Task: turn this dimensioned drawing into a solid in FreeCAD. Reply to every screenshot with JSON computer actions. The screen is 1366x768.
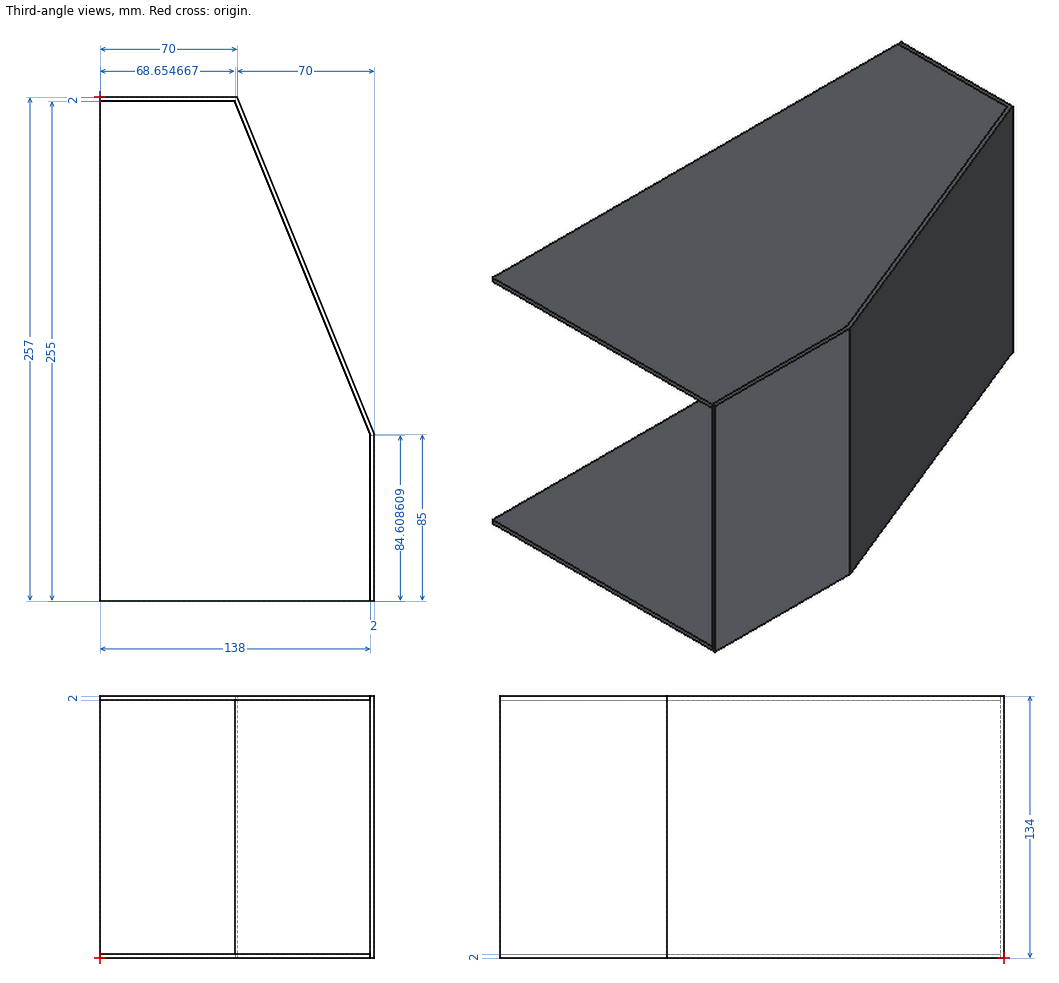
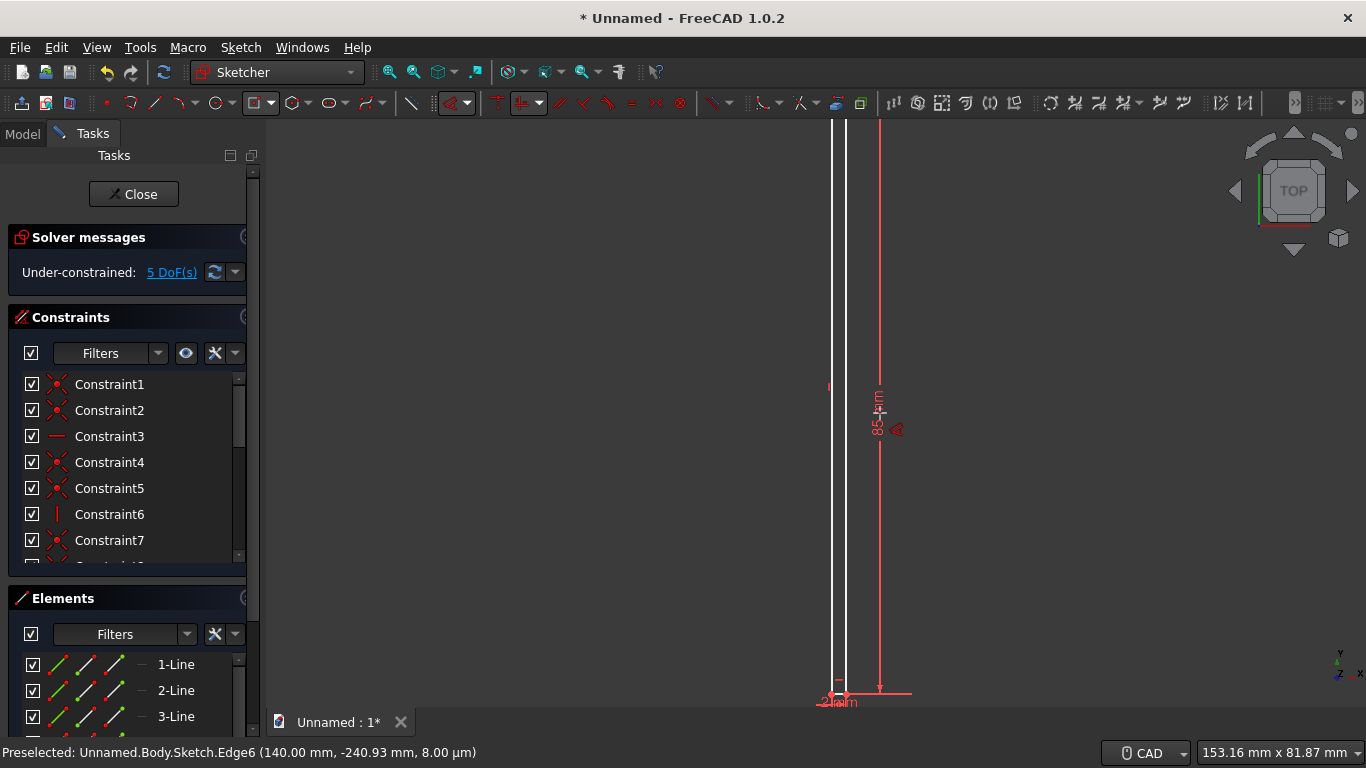
{"action": "scroll", "coordinate": [850, 576], "scroll_direction": "down", "scroll_amount": 8}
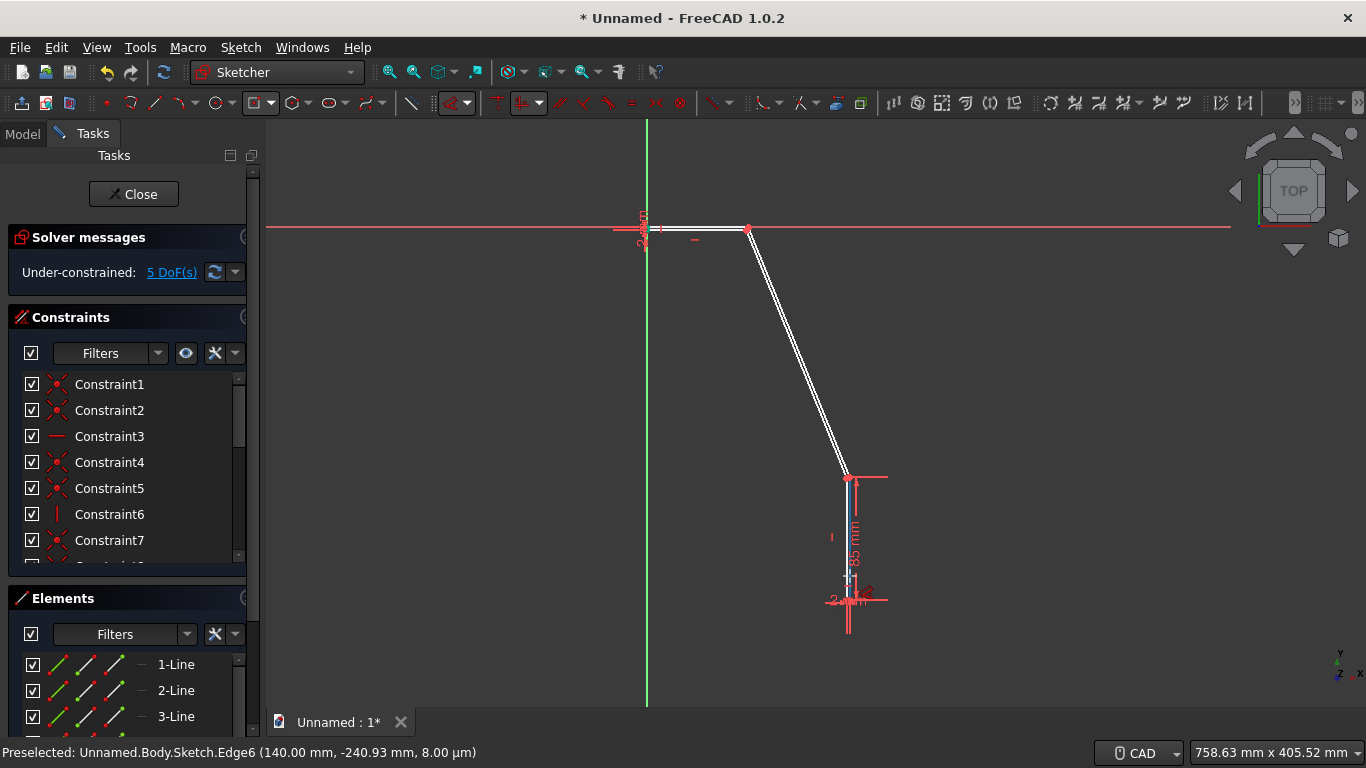
{"action": "scroll", "coordinate": [718, 227], "scroll_direction": "up", "scroll_amount": 8}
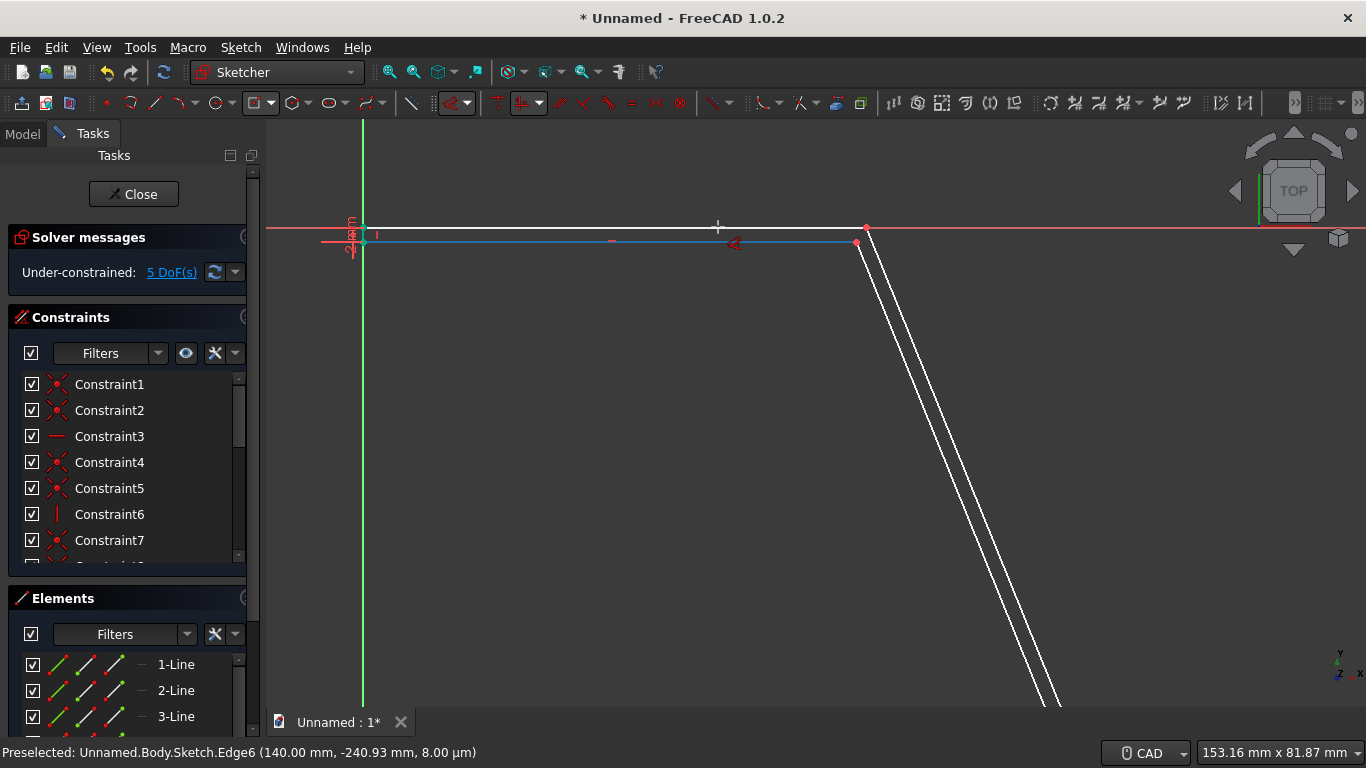
{"action": "left_click", "coordinate": [715, 228]}
{"action": "left_click", "coordinate": [615, 194]}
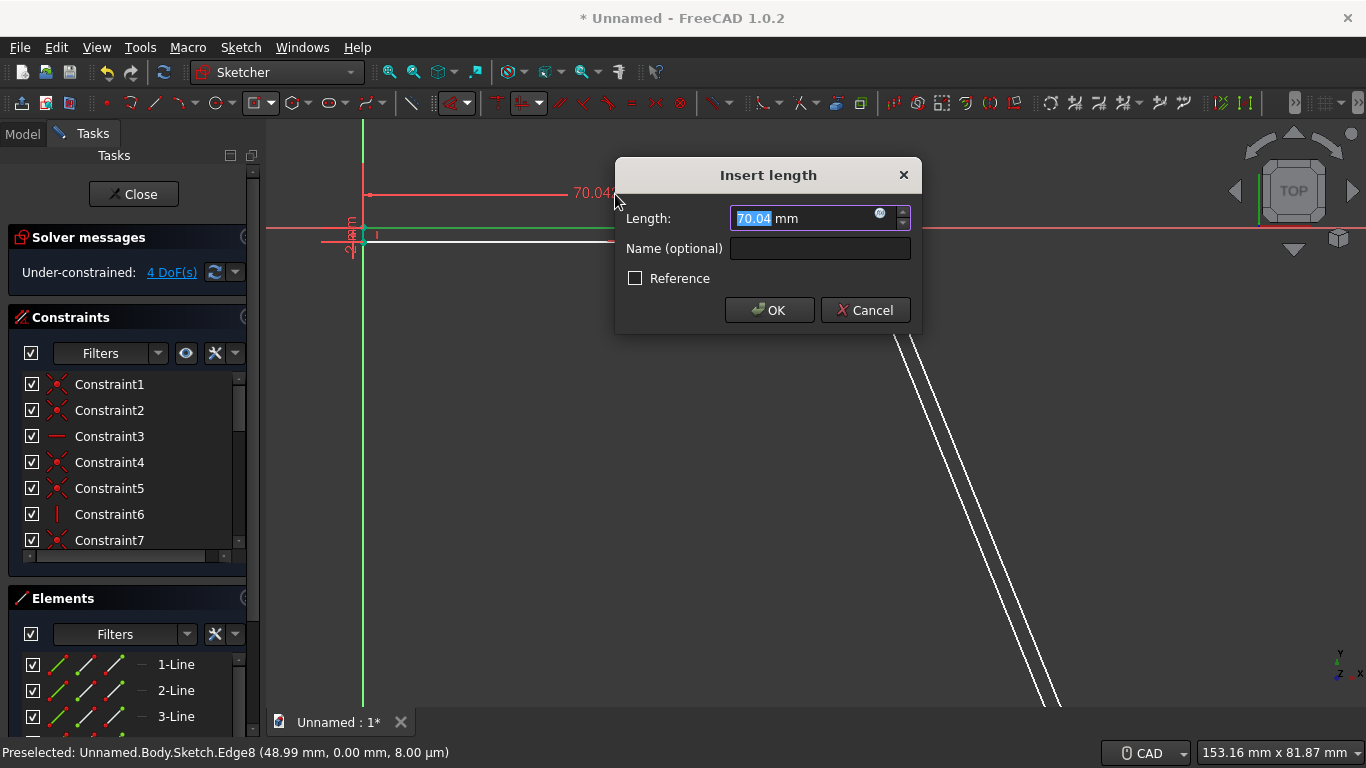
{"action": "type", "text": "70"}
{"action": "key", "text": "Return"}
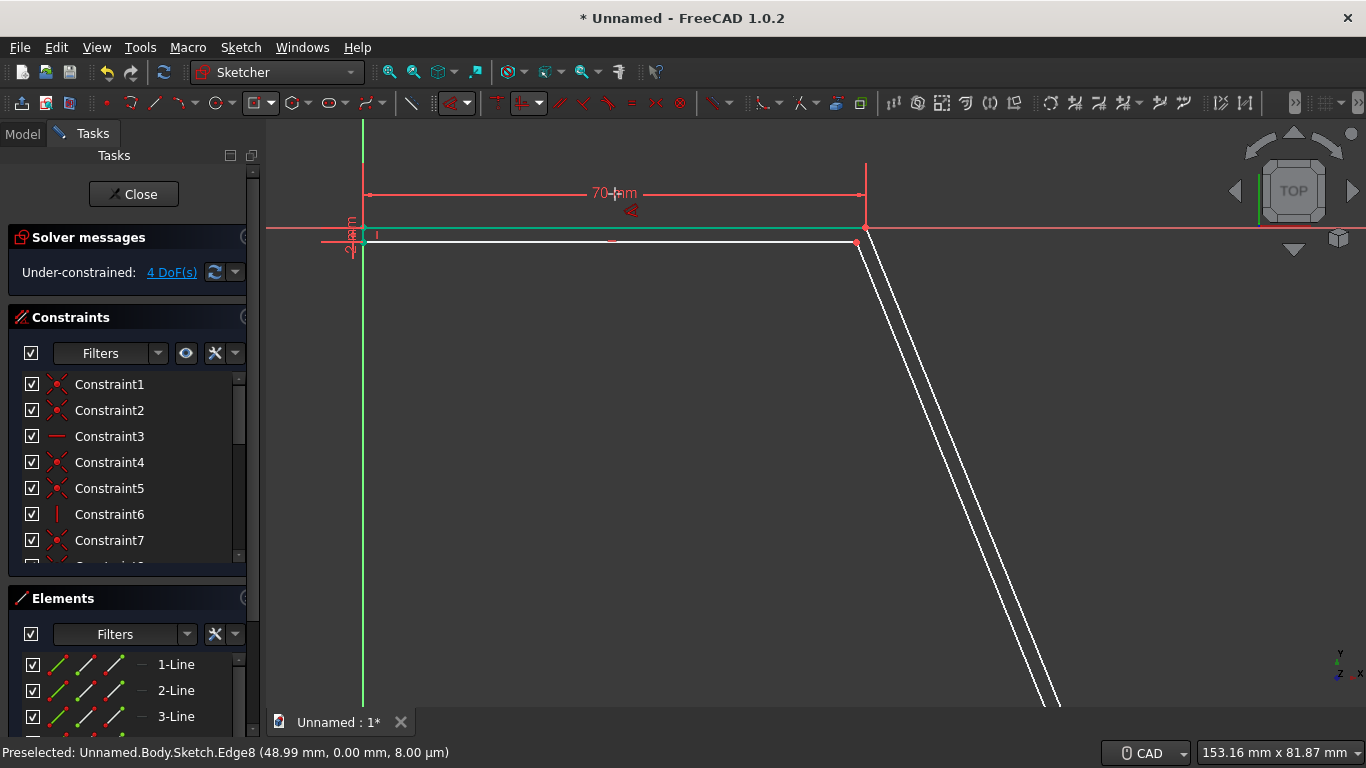
{"action": "left_click", "coordinate": [1017, 599]}
{"action": "left_click", "coordinate": [1033, 194]}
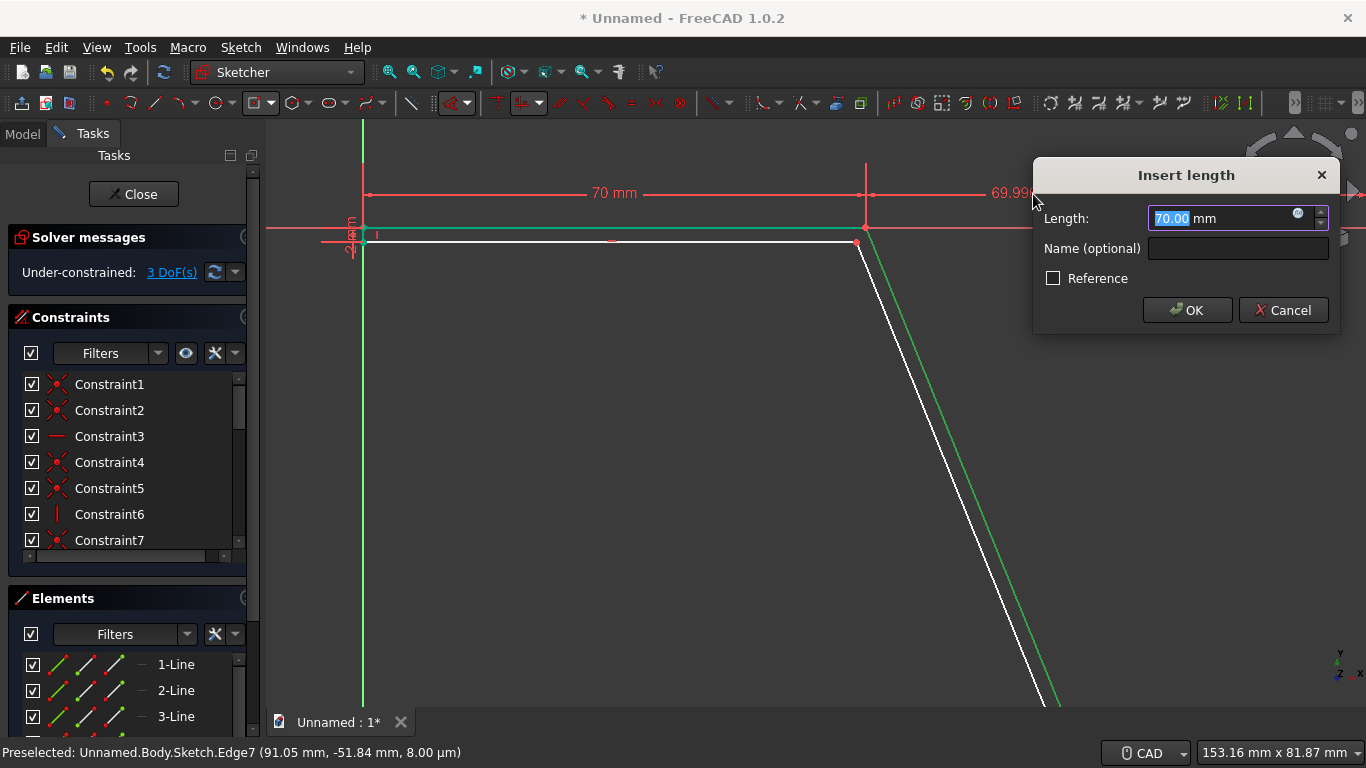
{"action": "type", "text": "70"}
{"action": "key", "text": "Return"}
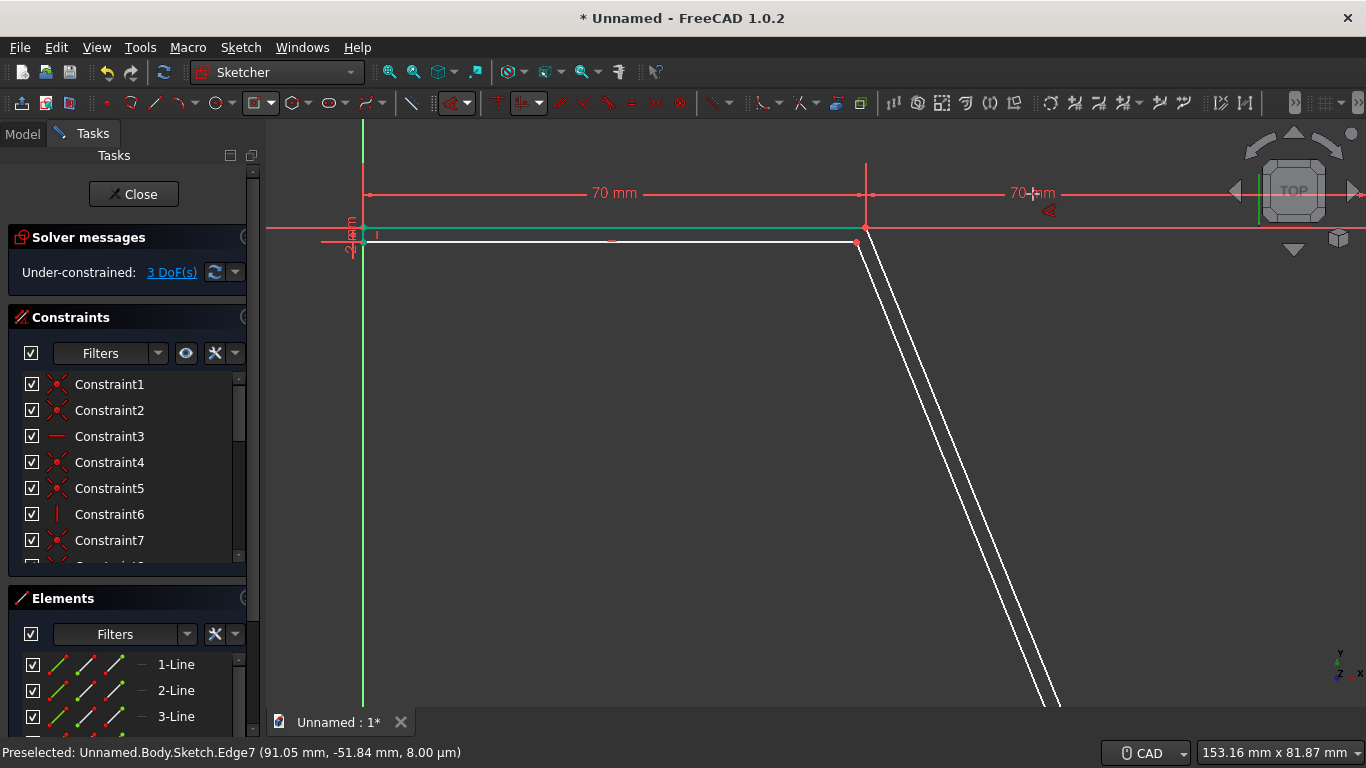
{"action": "scroll", "coordinate": [718, 226], "scroll_direction": "down", "scroll_amount": 8}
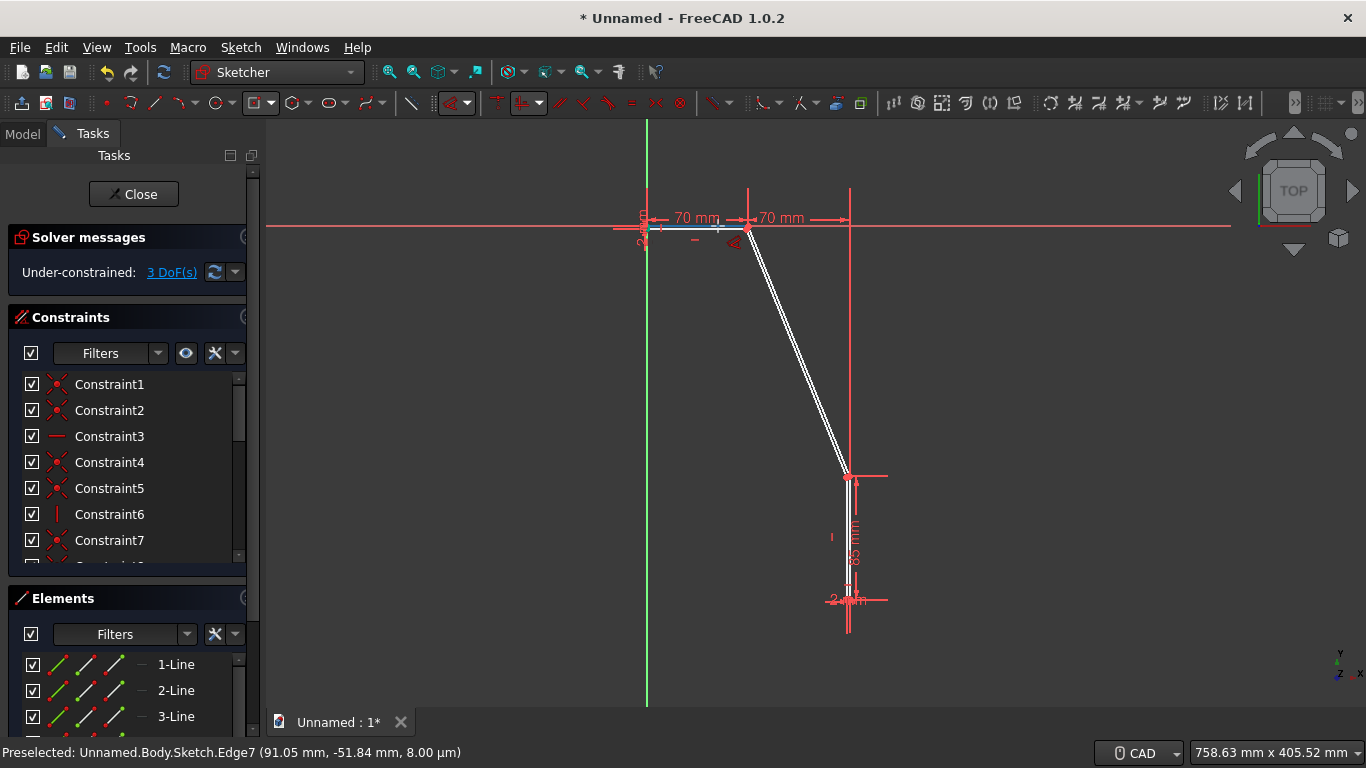
{"action": "scroll", "coordinate": [847, 600], "scroll_direction": "up", "scroll_amount": 8}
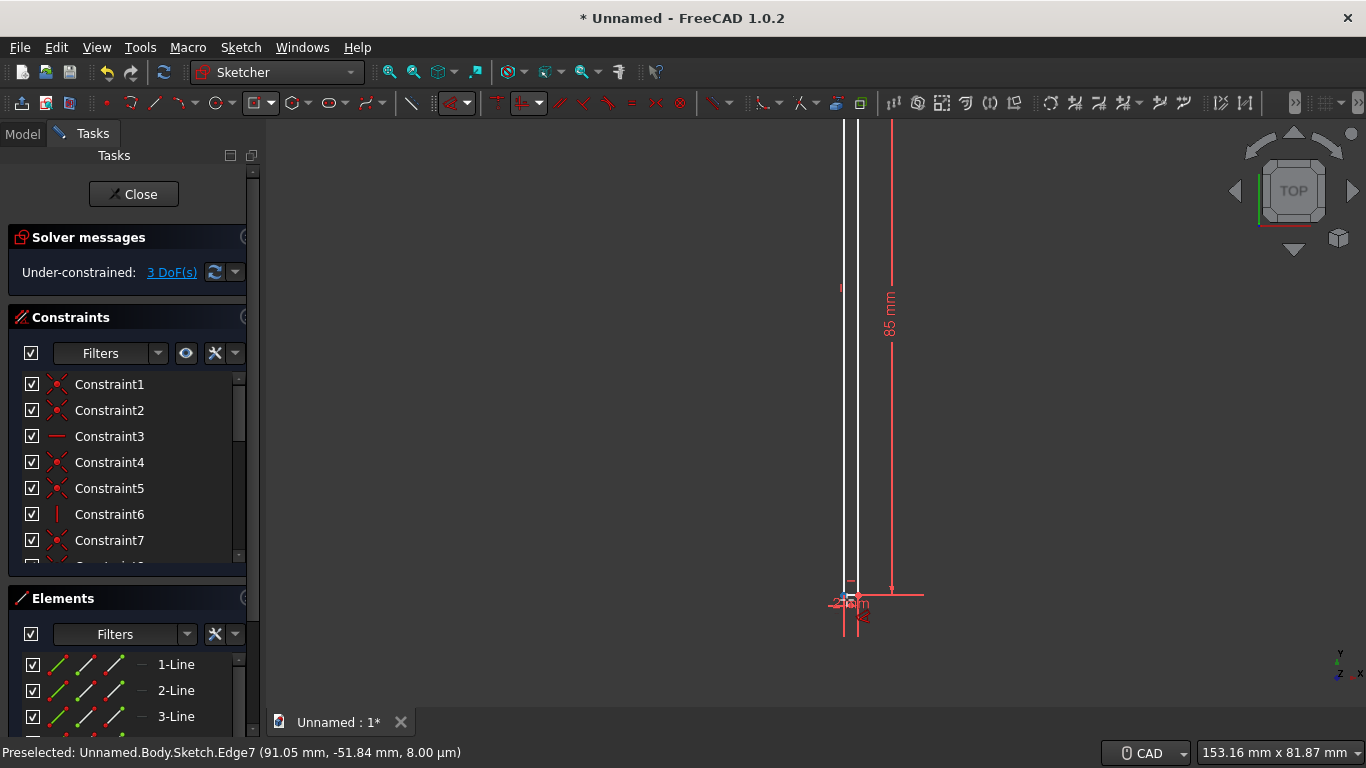
{"action": "left_click", "coordinate": [844, 595]}
{"action": "left_click", "coordinate": [878, 371]}